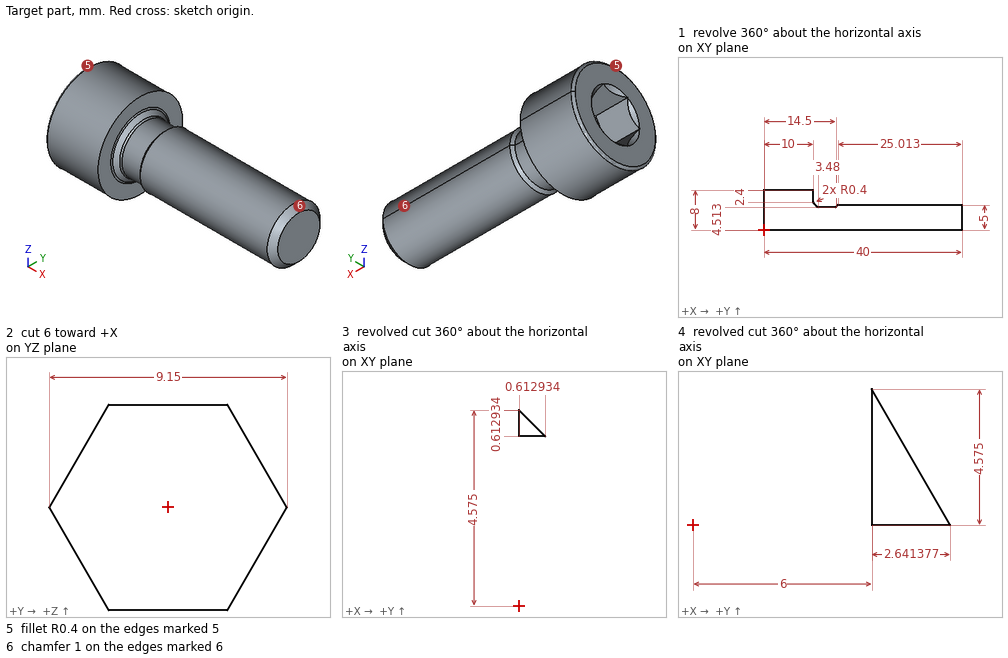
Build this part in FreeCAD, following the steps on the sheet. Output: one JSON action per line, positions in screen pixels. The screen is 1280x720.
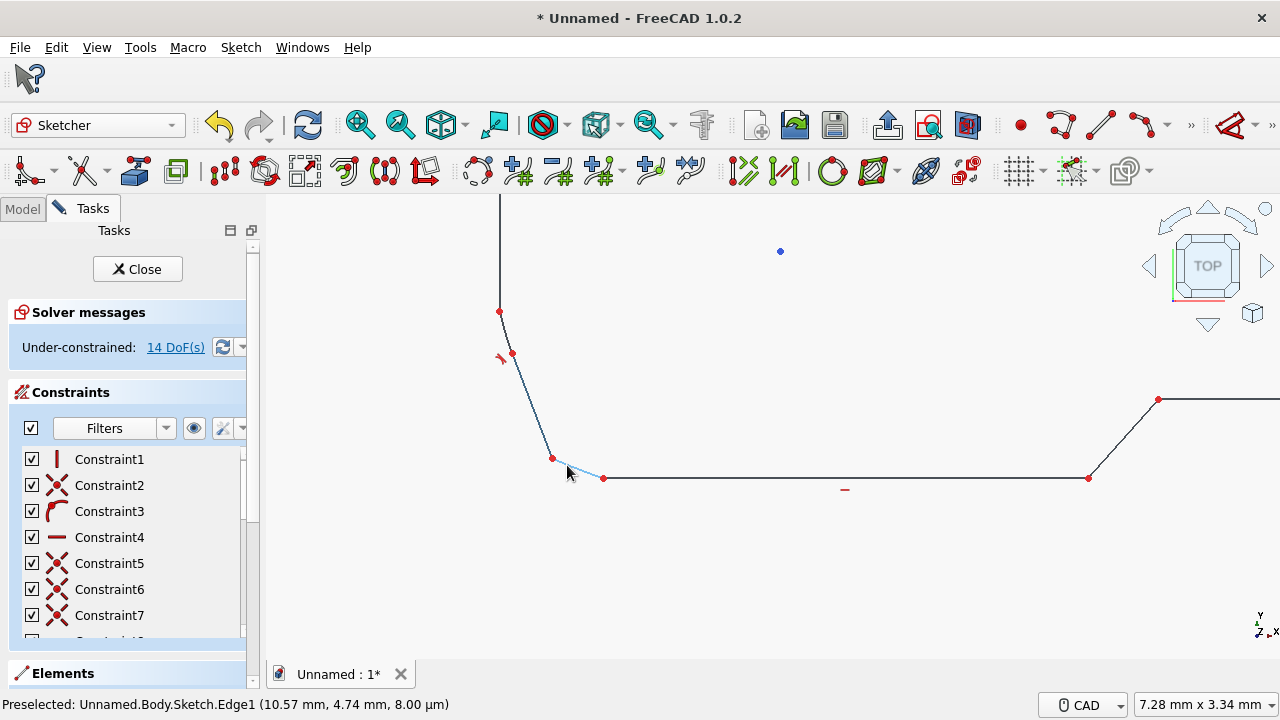
{"action": "left_click", "coordinate": [567, 465]}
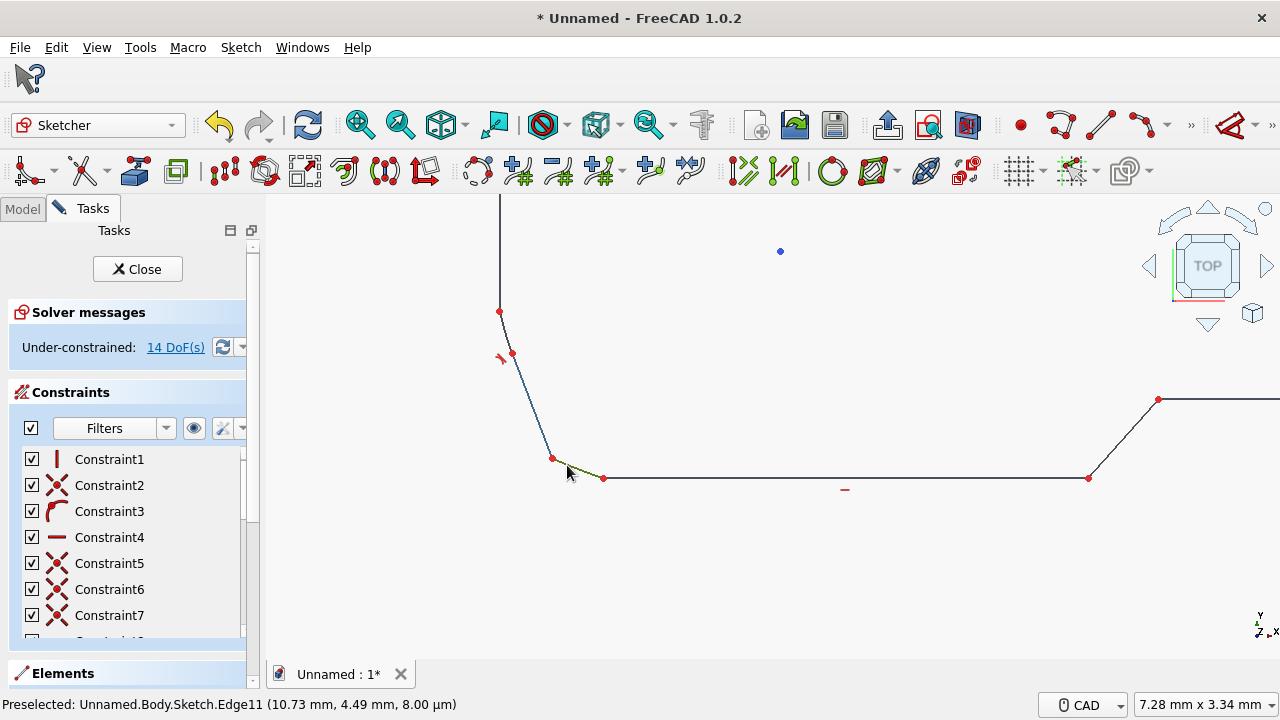
{"action": "key", "text": "t"}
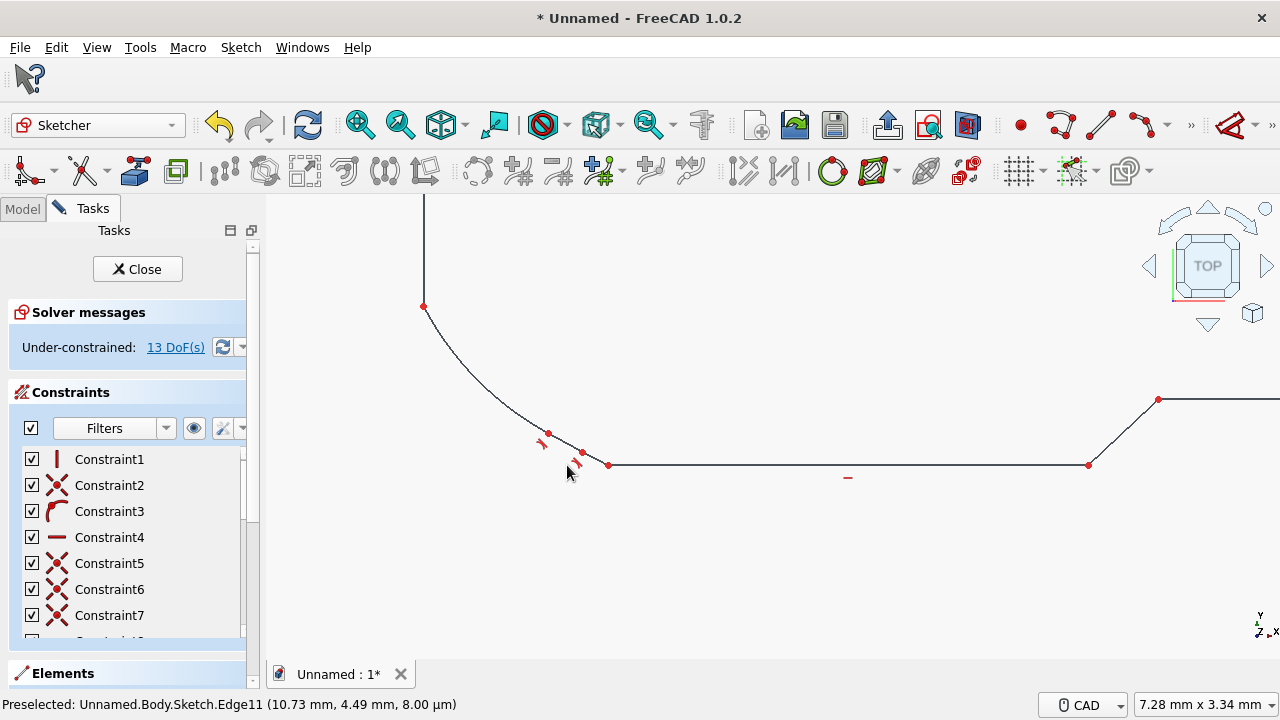
{"action": "scroll", "coordinate": [561, 413], "scroll_direction": "down", "scroll_amount": 11}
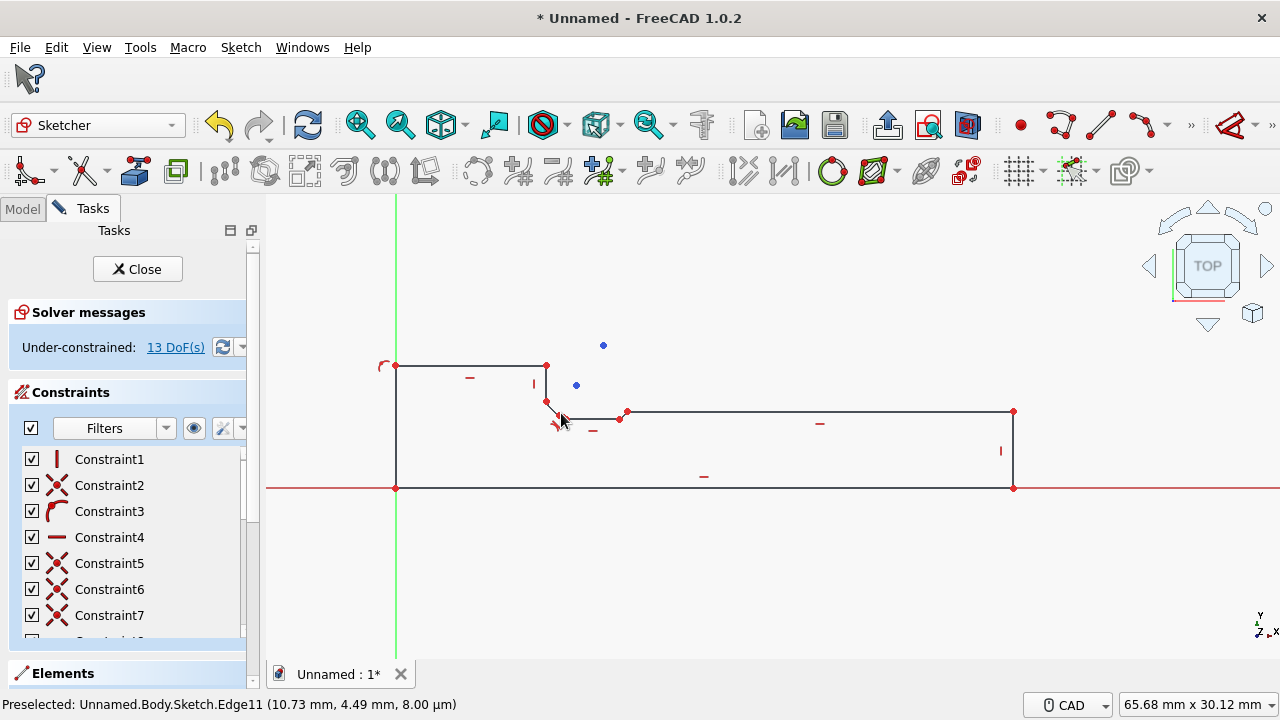
{"action": "scroll", "coordinate": [546, 394], "scroll_direction": "up", "scroll_amount": 4}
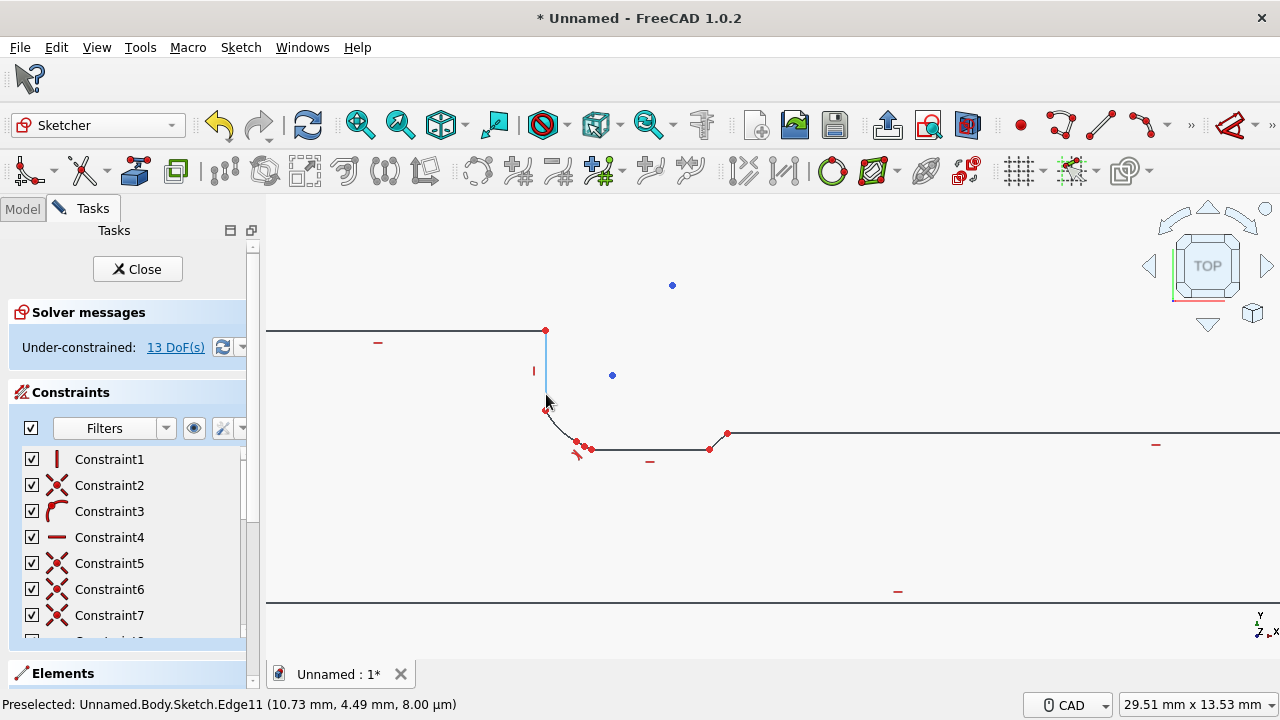
{"action": "left_click", "coordinate": [546, 395]}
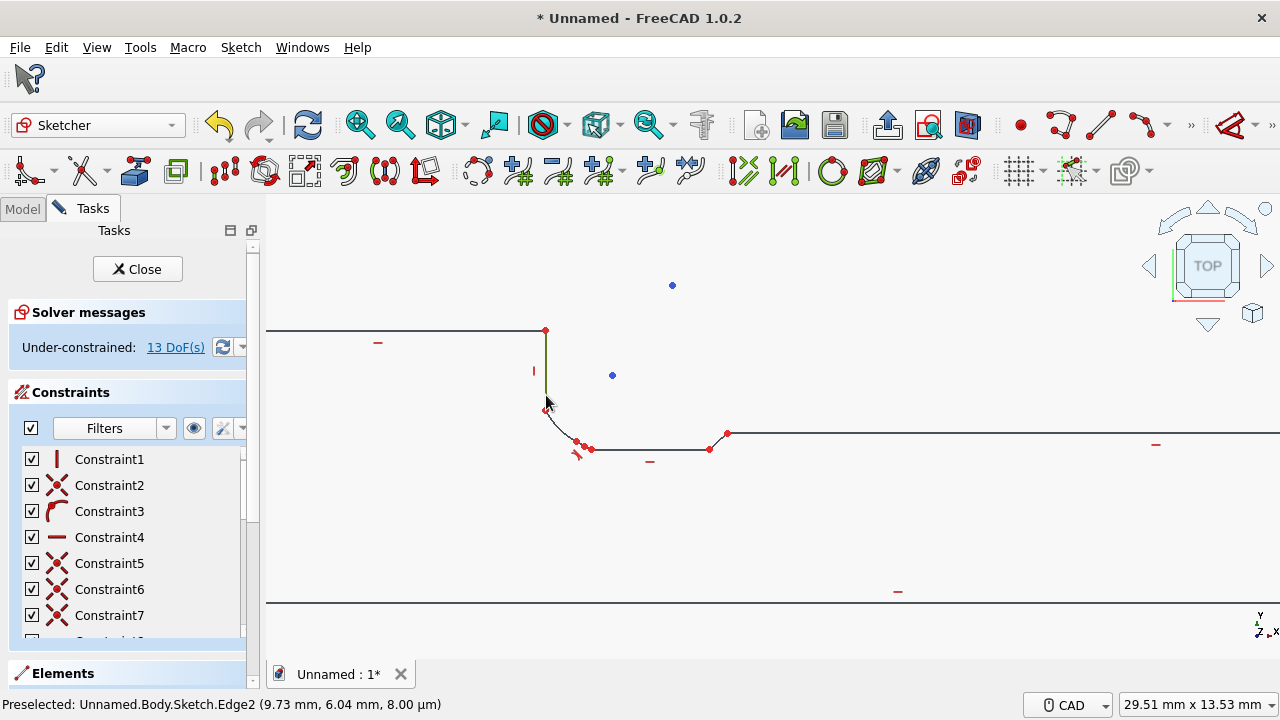
{"action": "left_click", "coordinate": [553, 422]}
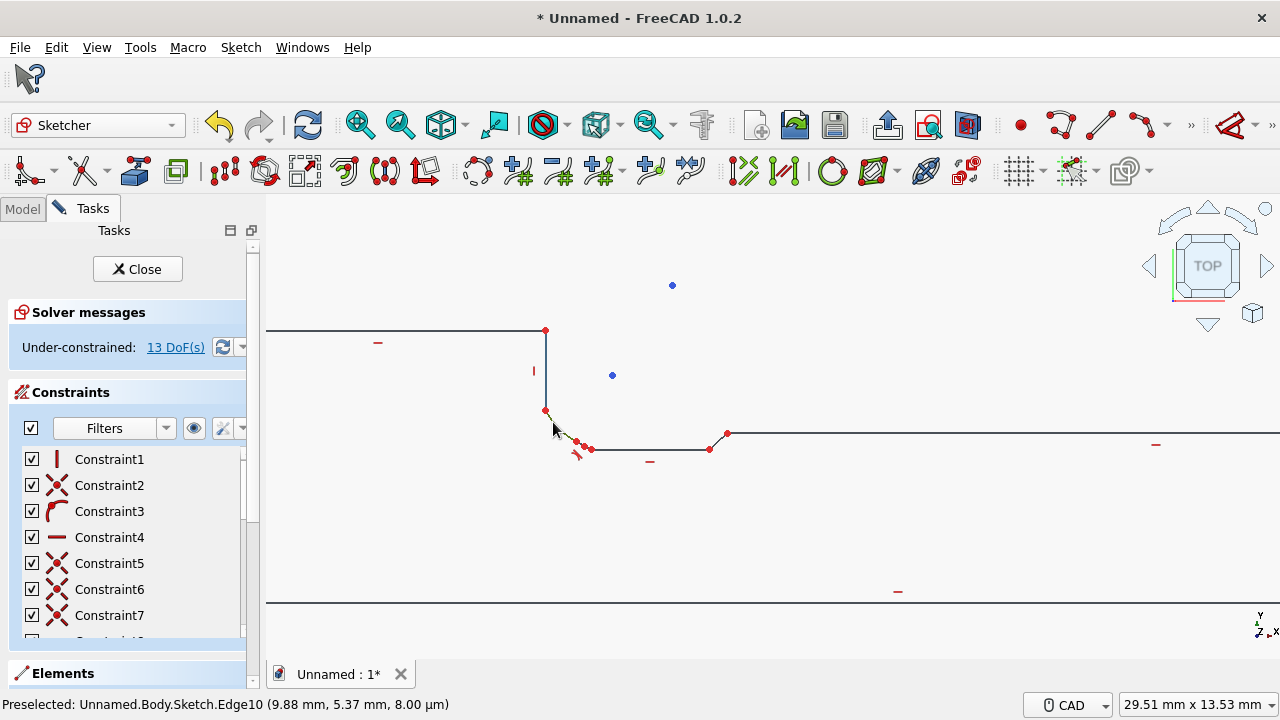
{"action": "key", "text": "t"}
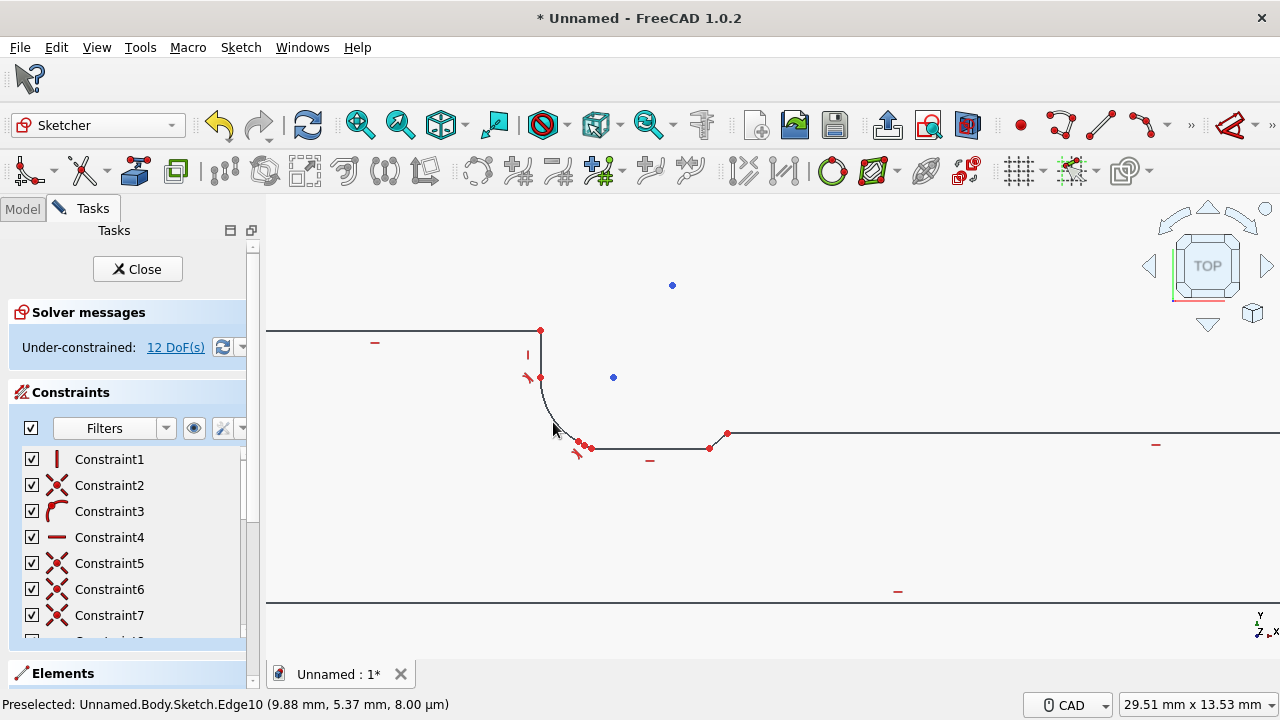
{"action": "left_click", "coordinate": [674, 449]}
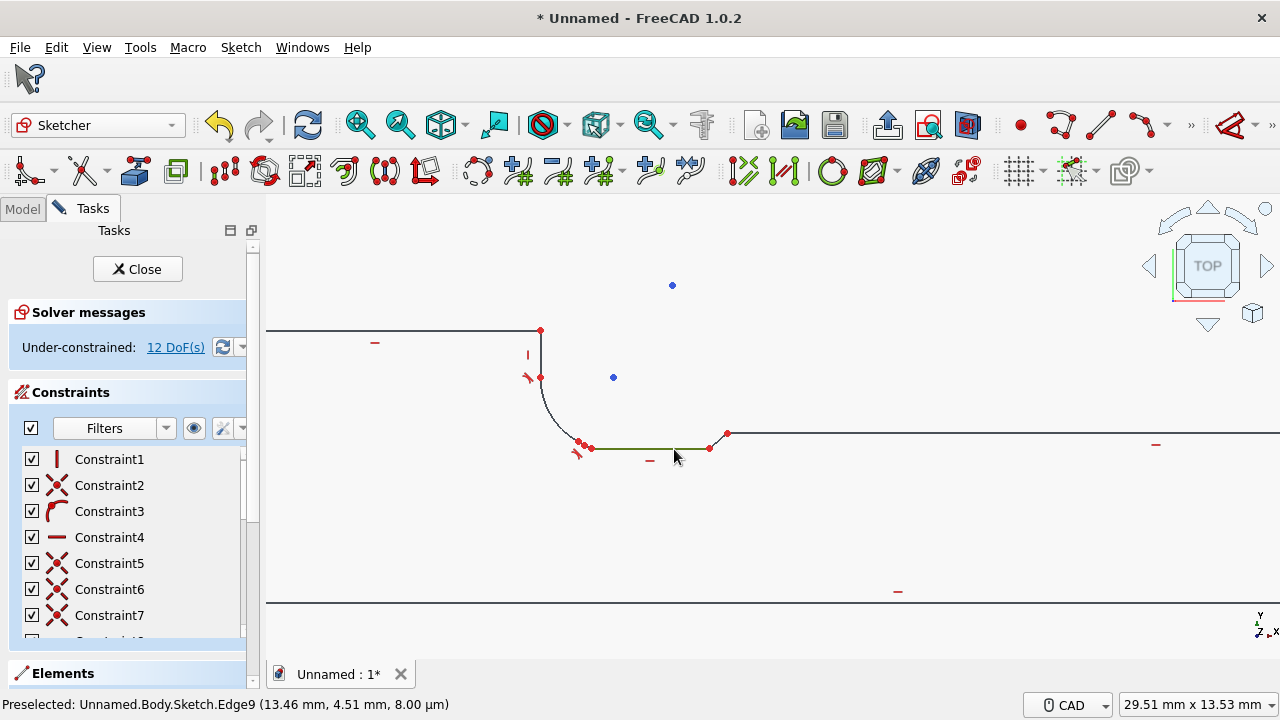
{"action": "scroll", "coordinate": [588, 447], "scroll_direction": "up", "scroll_amount": 7}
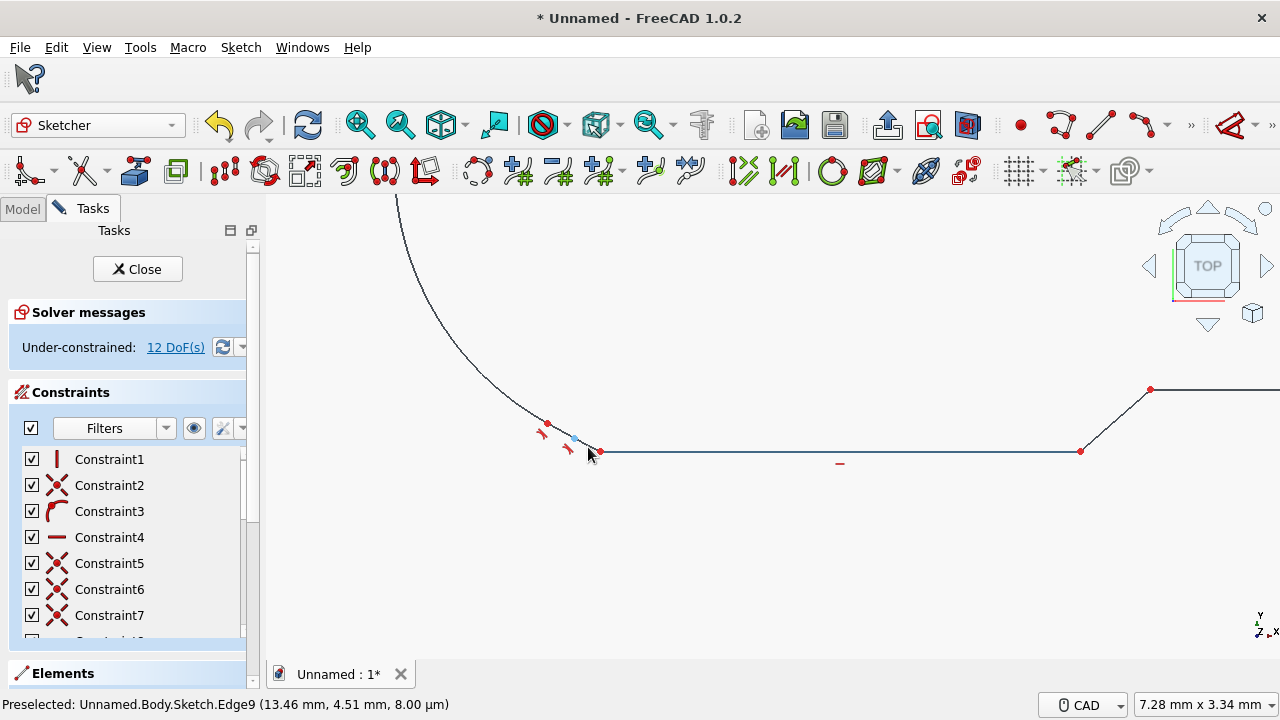
{"action": "left_click", "coordinate": [587, 445]}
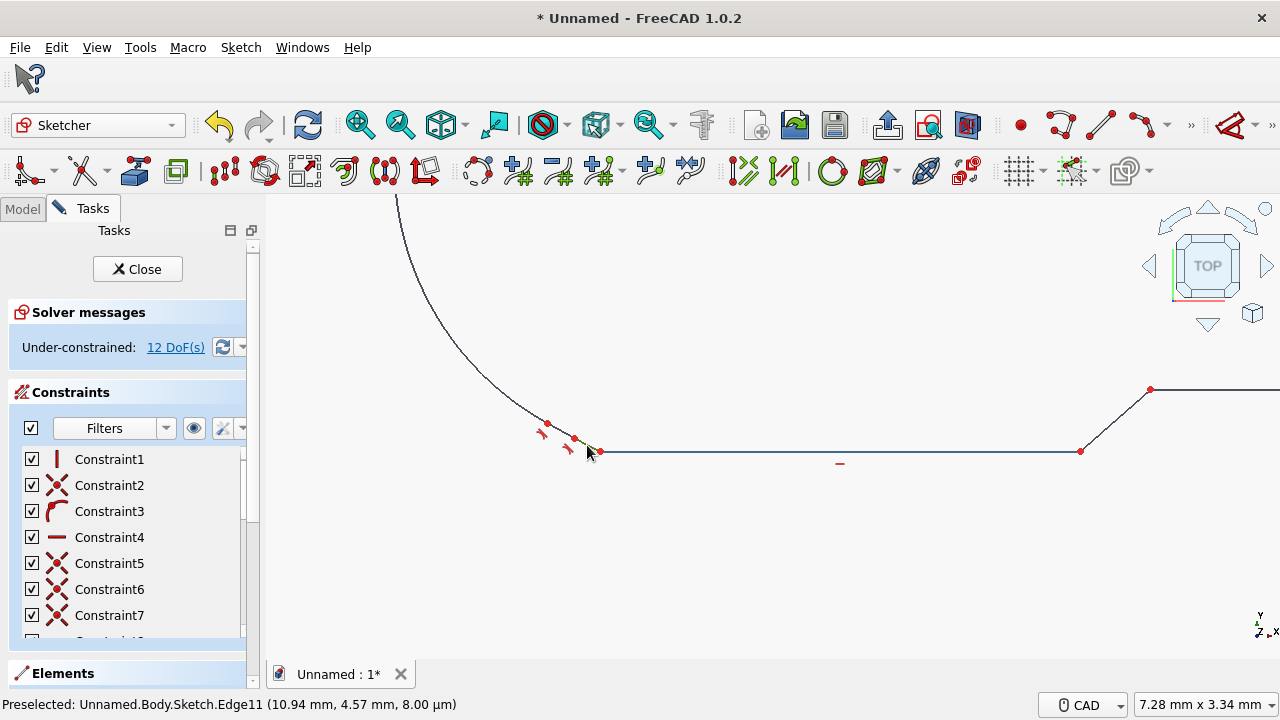
{"action": "key", "text": "t"}